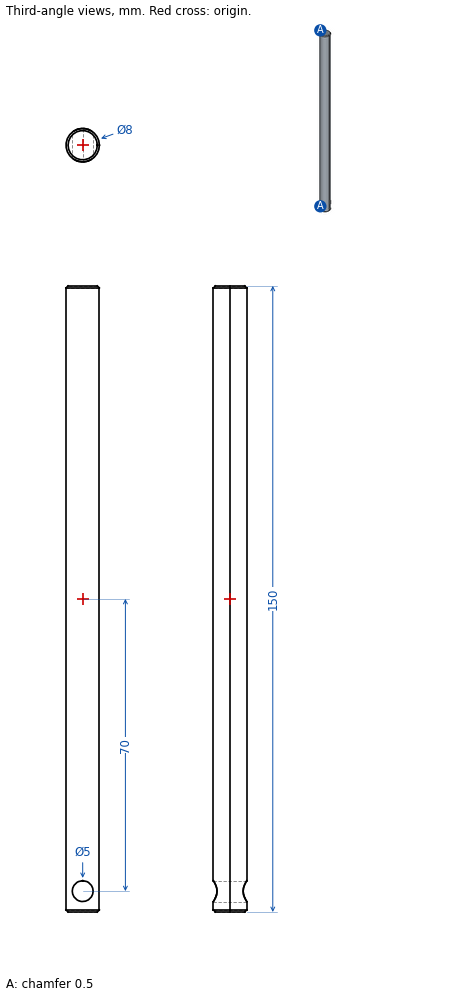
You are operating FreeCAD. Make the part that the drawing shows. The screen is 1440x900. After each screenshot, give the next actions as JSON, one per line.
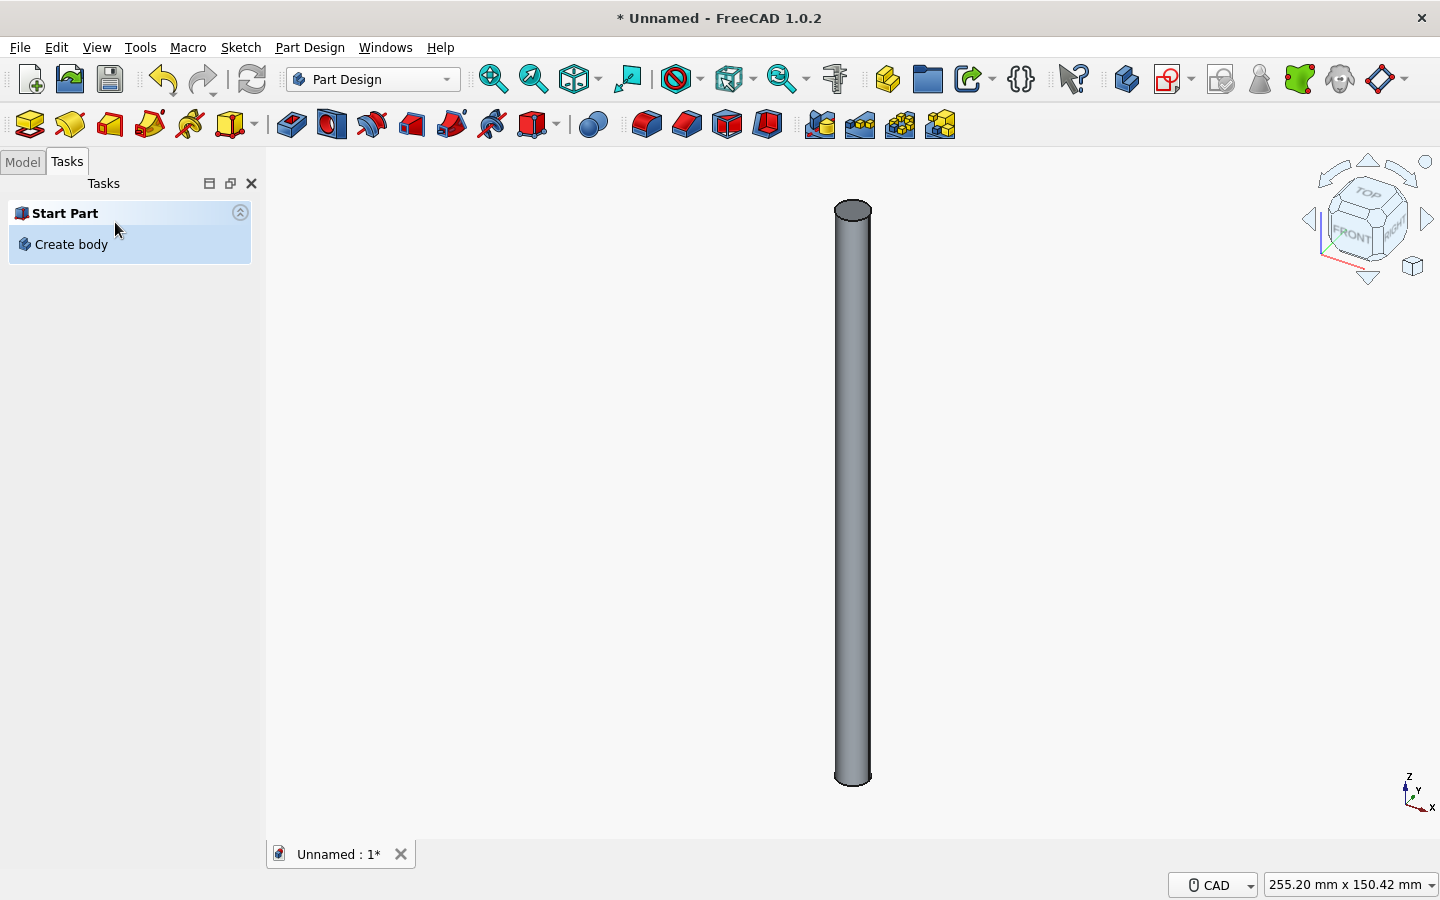
{"action": "left_click", "coordinate": [1168, 80]}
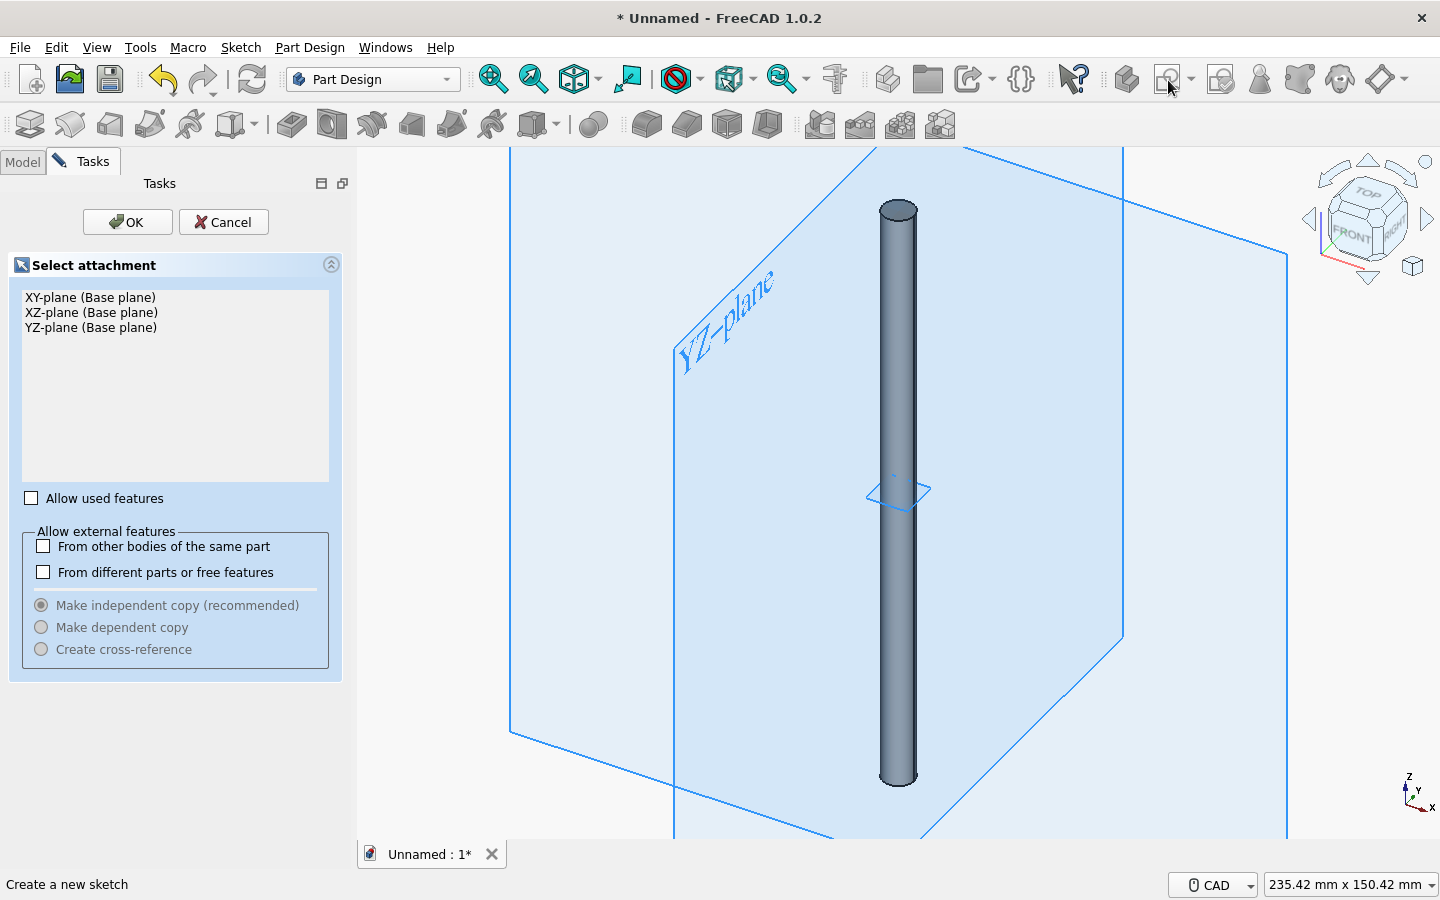
{"action": "left_click", "coordinate": [82, 312]}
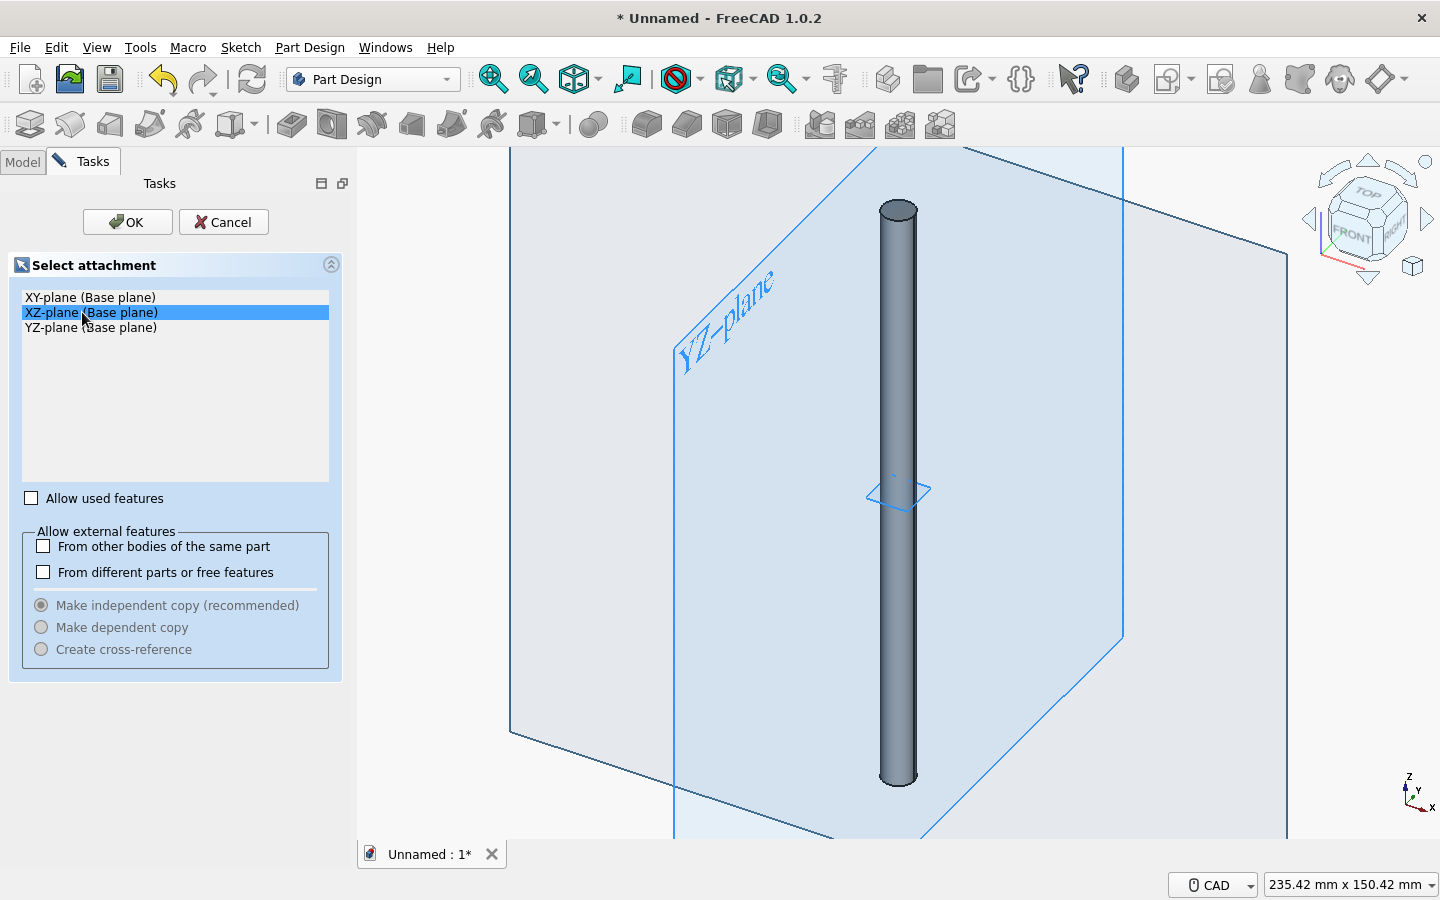
{"action": "left_click", "coordinate": [128, 222]}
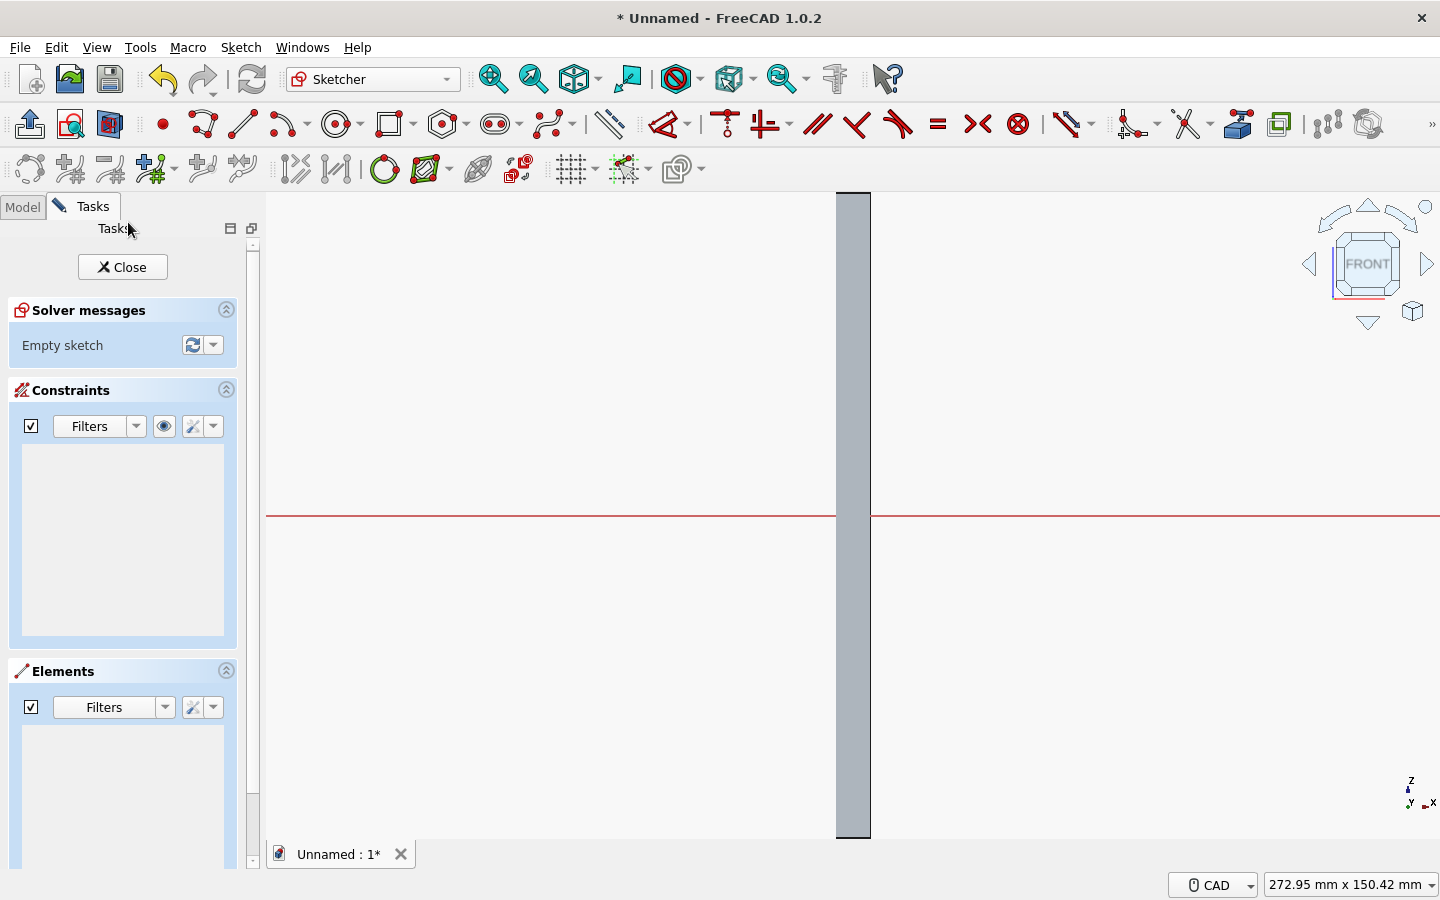
{"action": "left_click", "coordinate": [110, 124]}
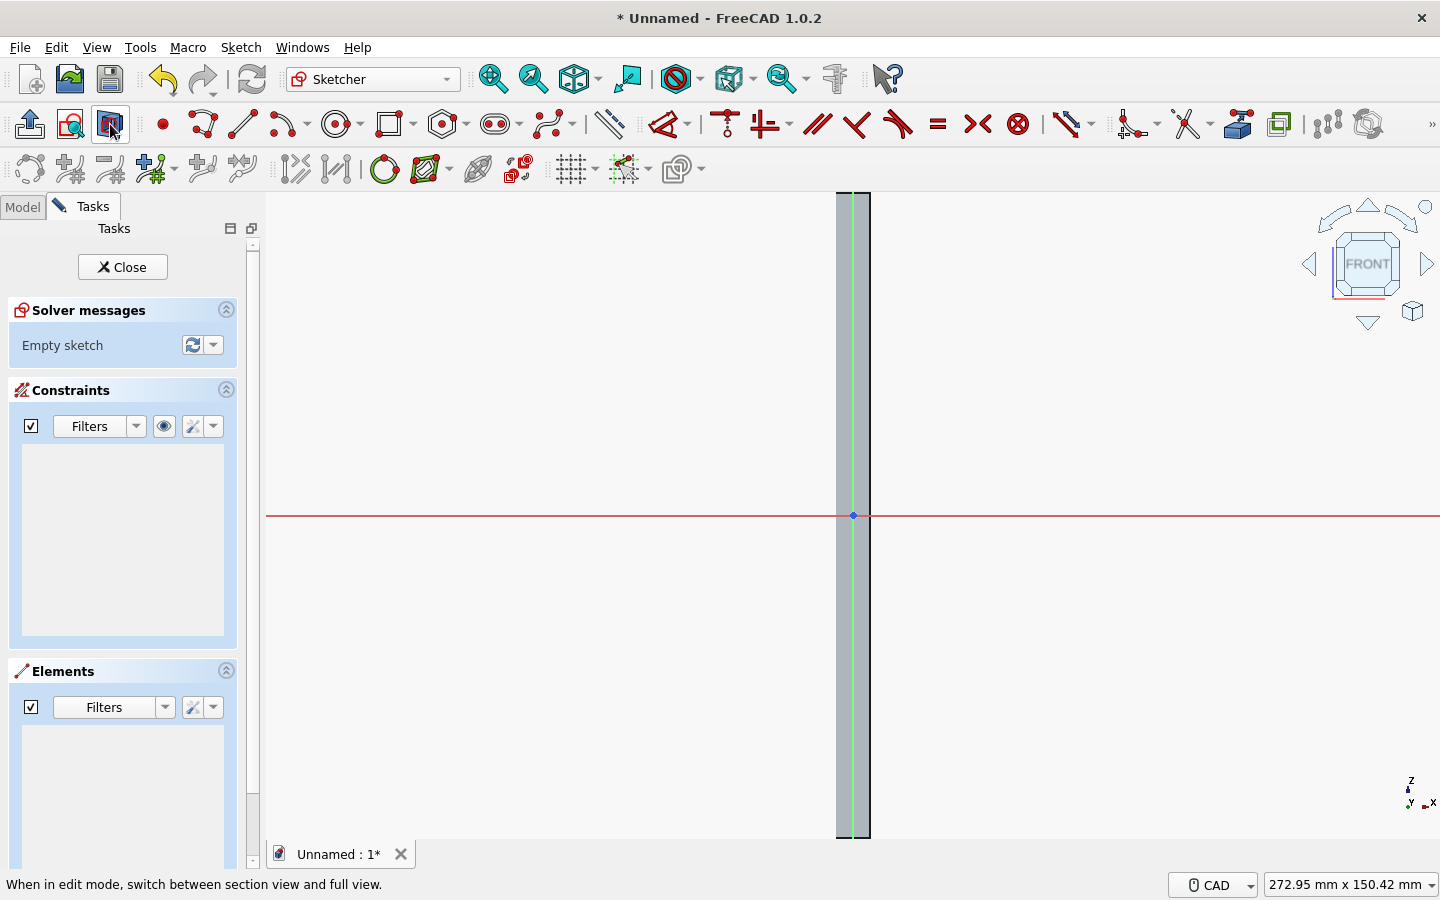
{"action": "scroll", "coordinate": [784, 516], "scroll_direction": "down", "scroll_amount": 5}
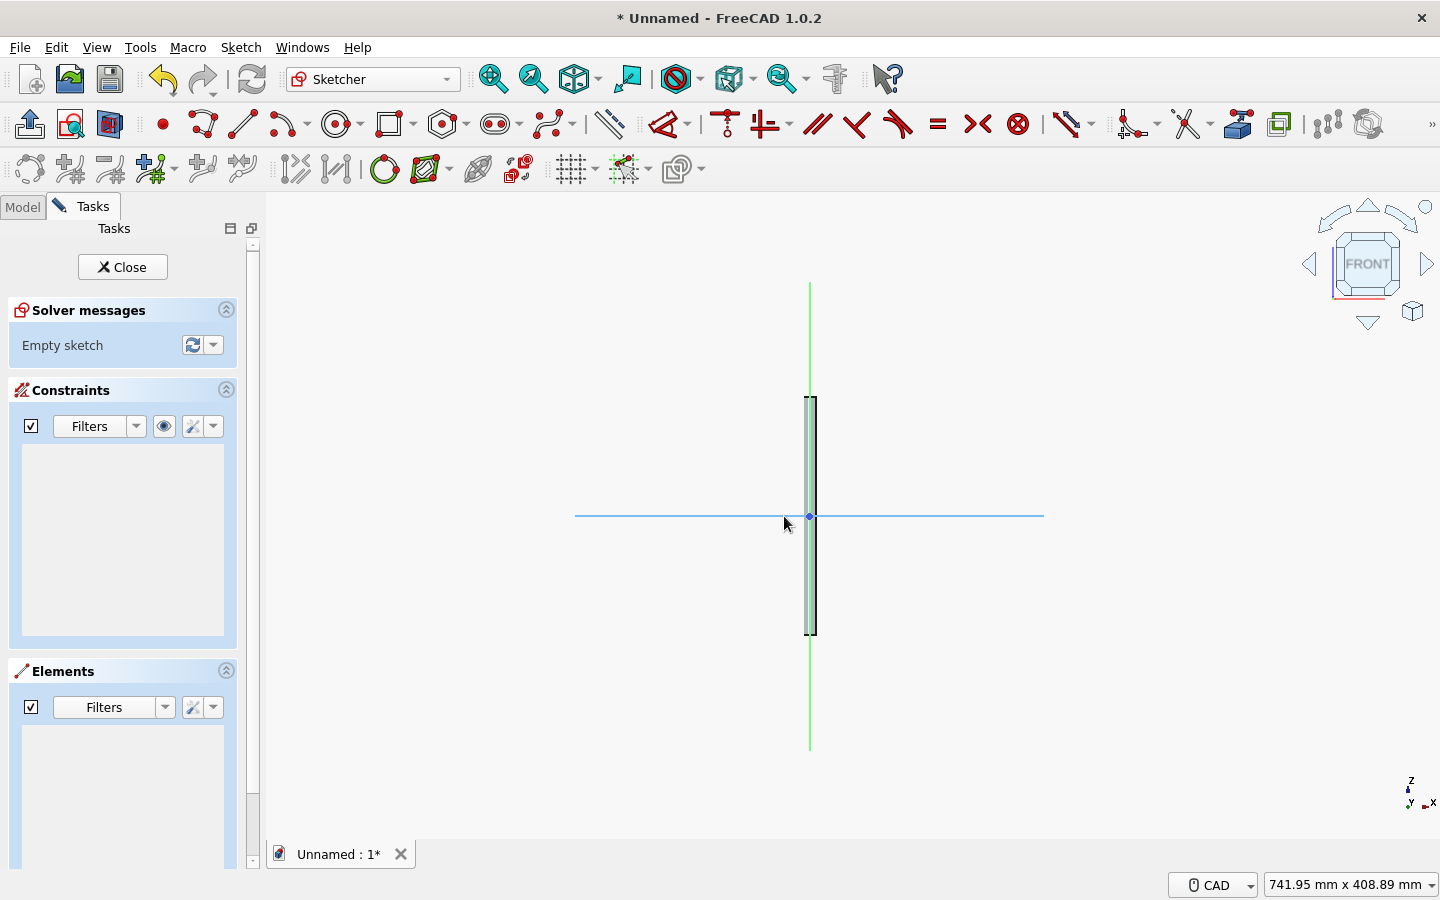
{"action": "scroll", "coordinate": [811, 633], "scroll_direction": "up", "scroll_amount": 15}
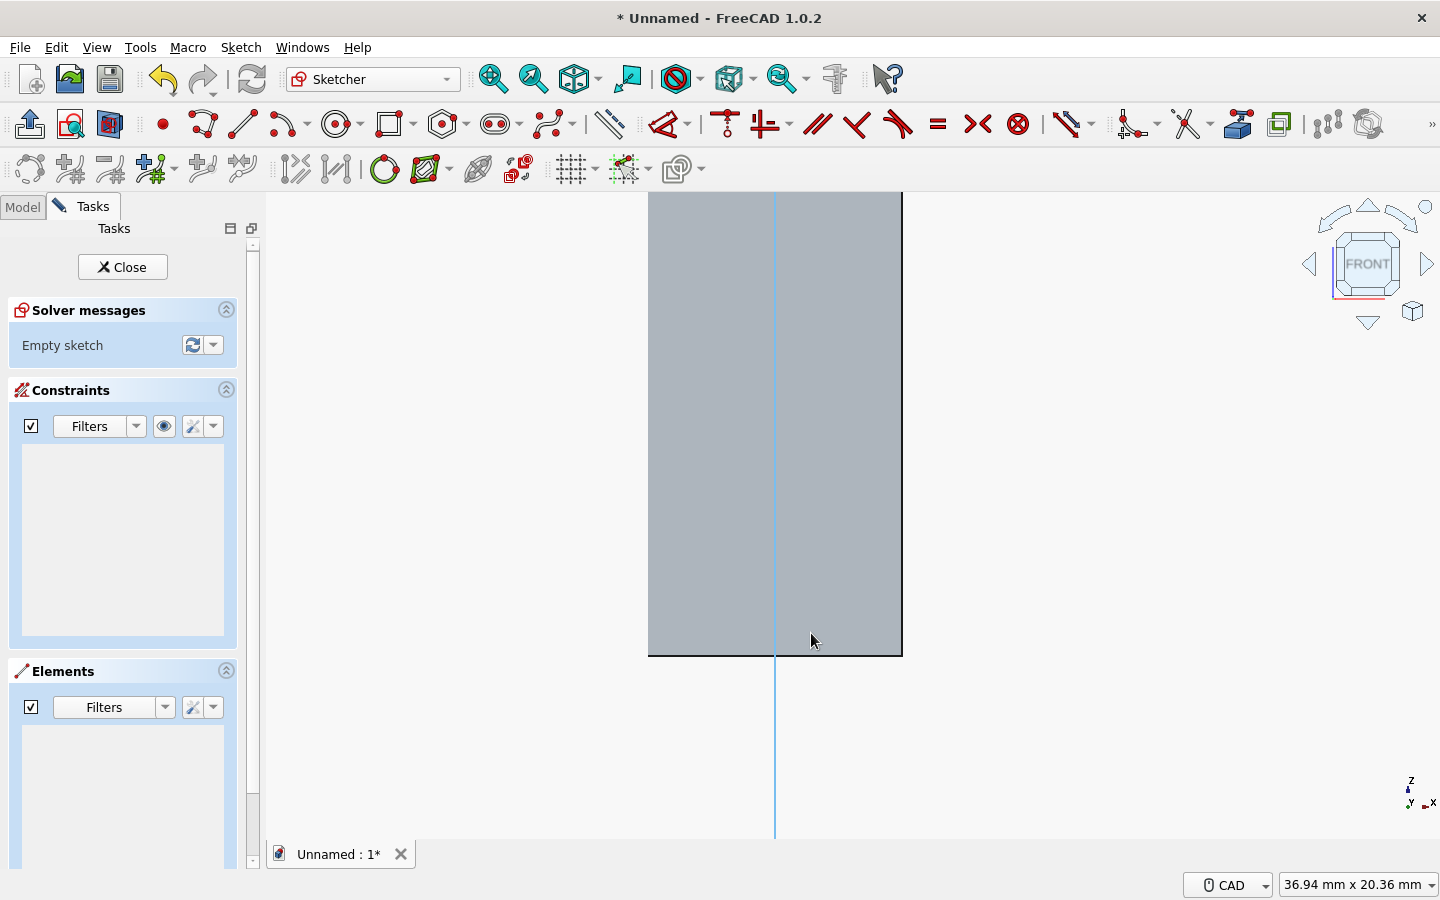
{"action": "scroll", "coordinate": [770, 487], "scroll_direction": "up", "scroll_amount": 5}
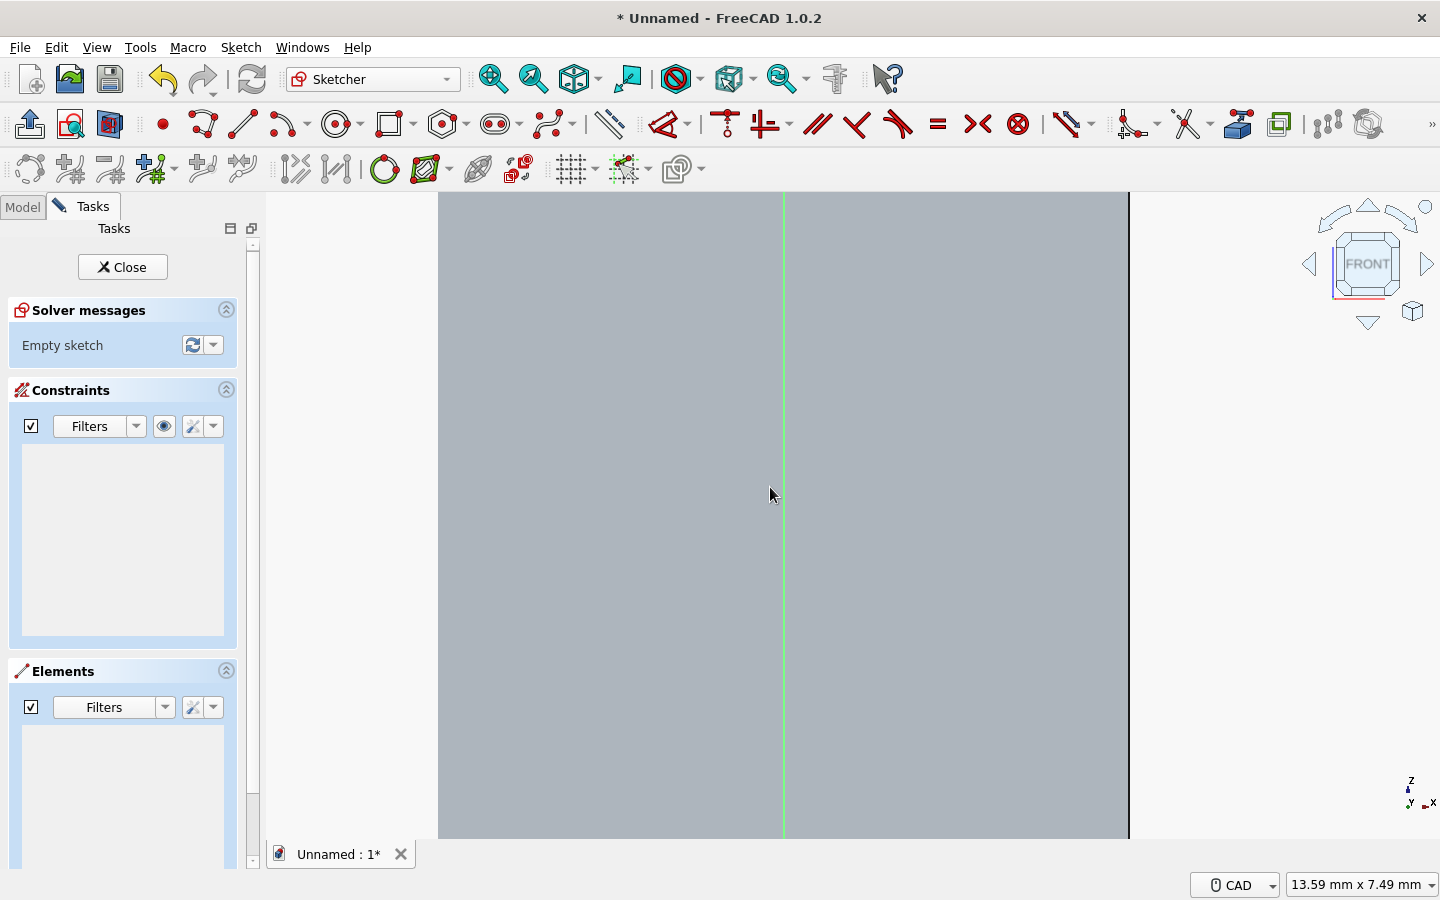
{"action": "left_click", "coordinate": [336, 124]}